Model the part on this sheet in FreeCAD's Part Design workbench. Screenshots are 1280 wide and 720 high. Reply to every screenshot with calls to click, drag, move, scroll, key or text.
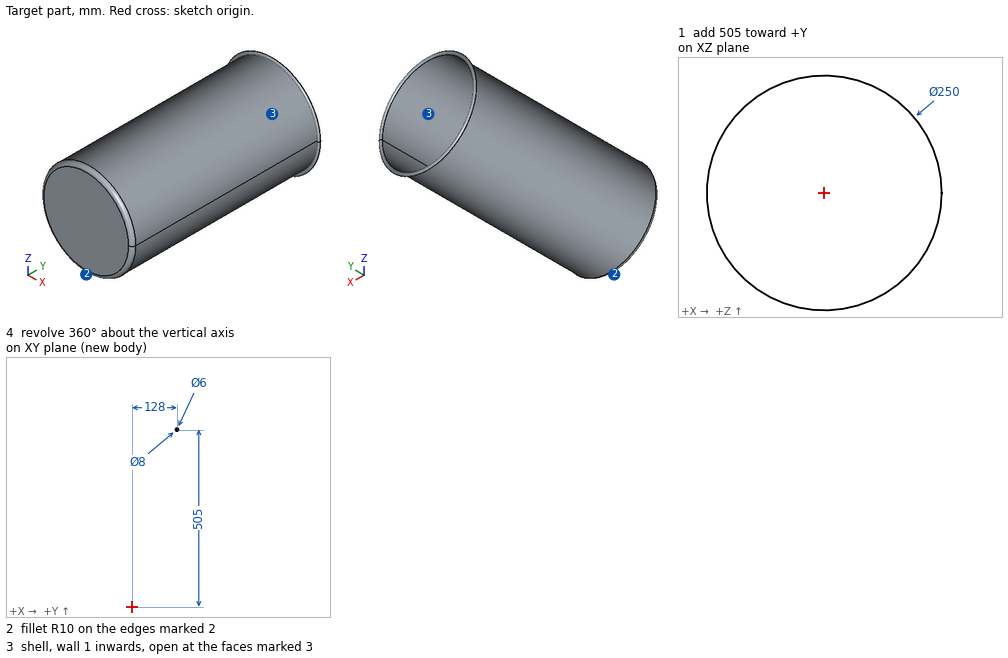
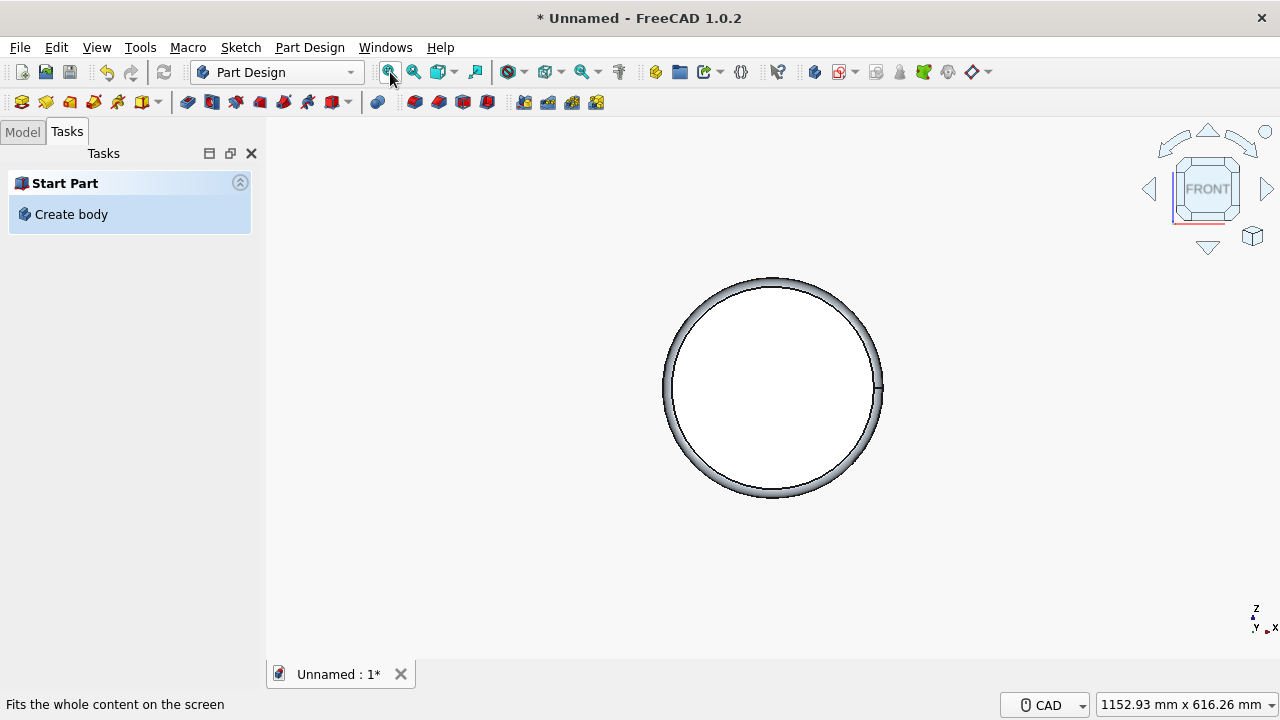
key(3)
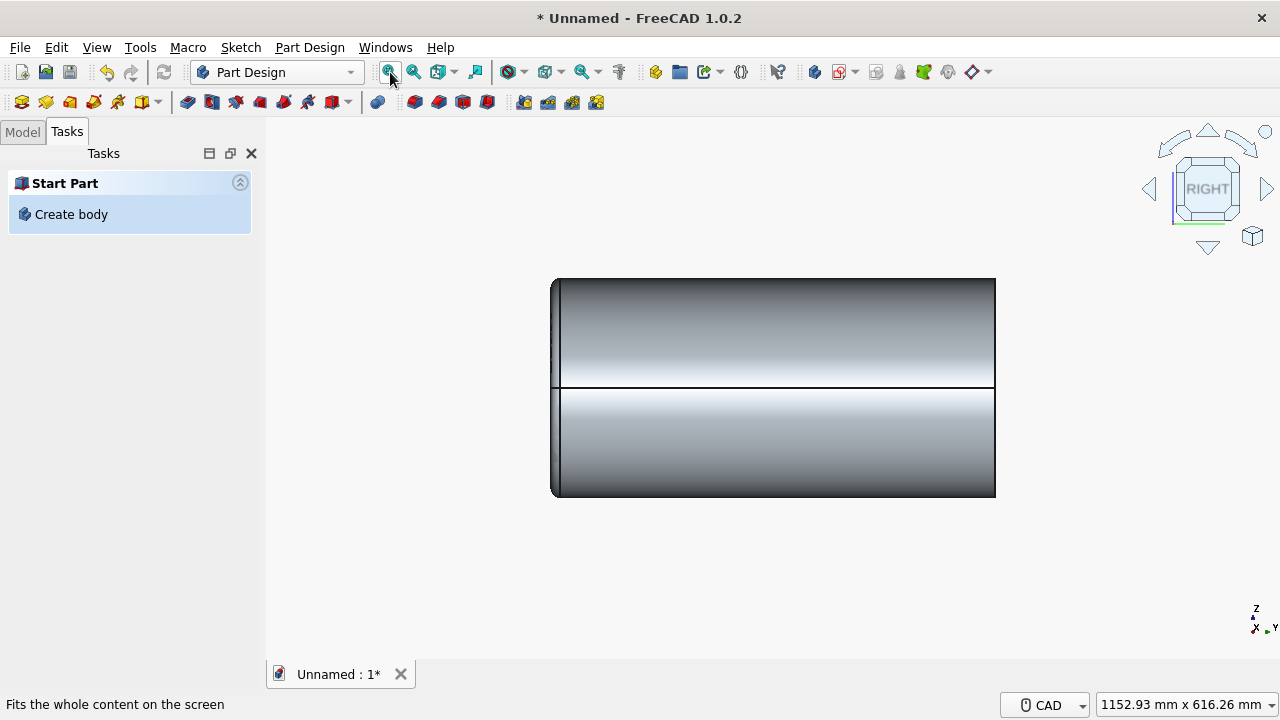
click(390, 72)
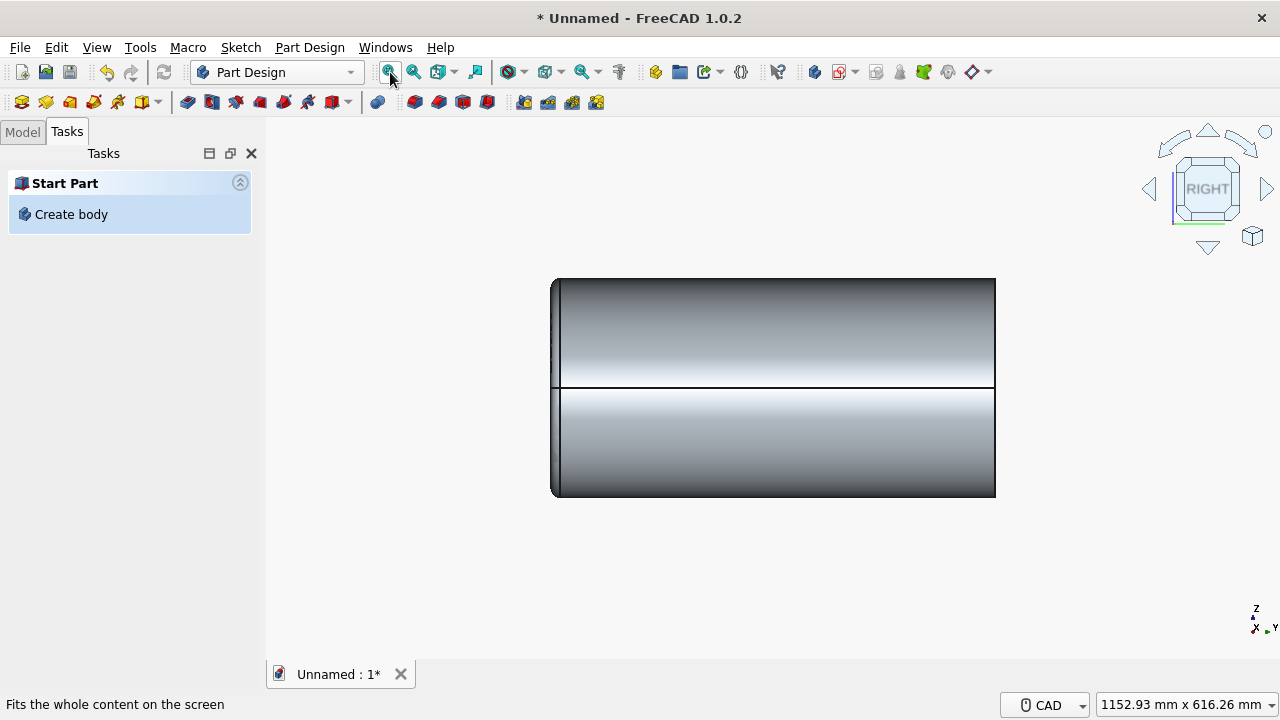
key(5)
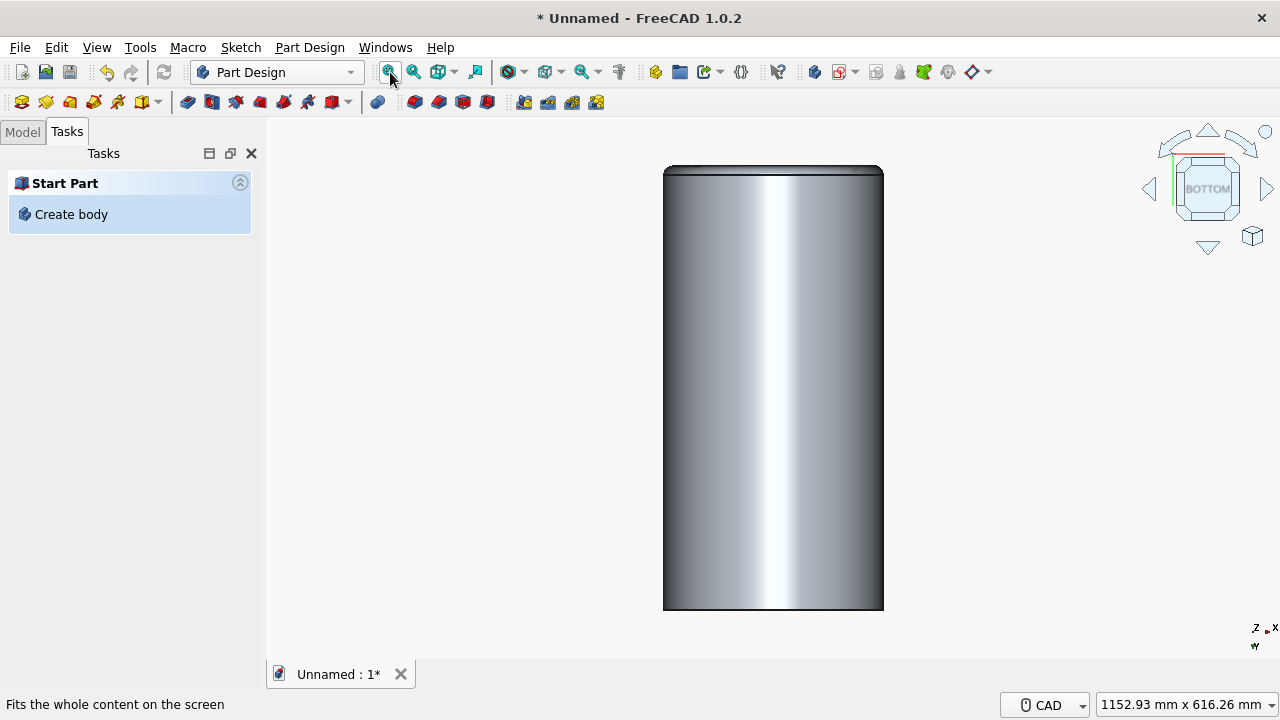
key(4)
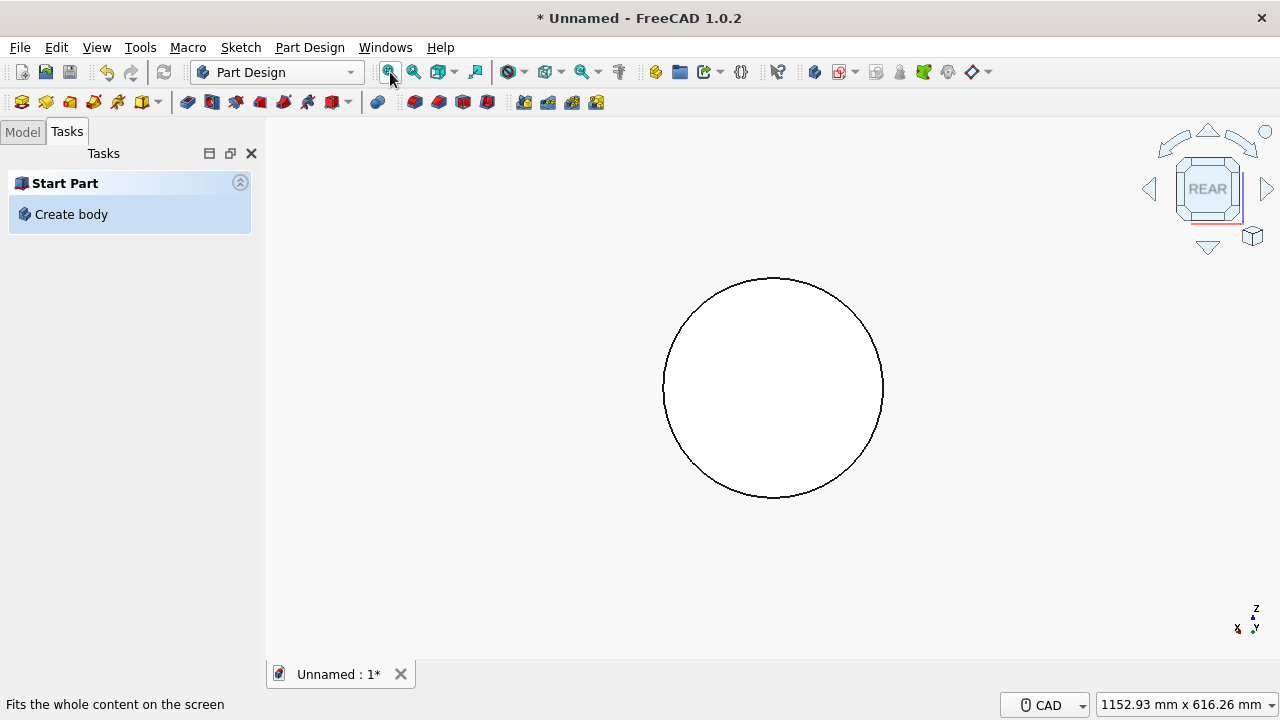
click(390, 72)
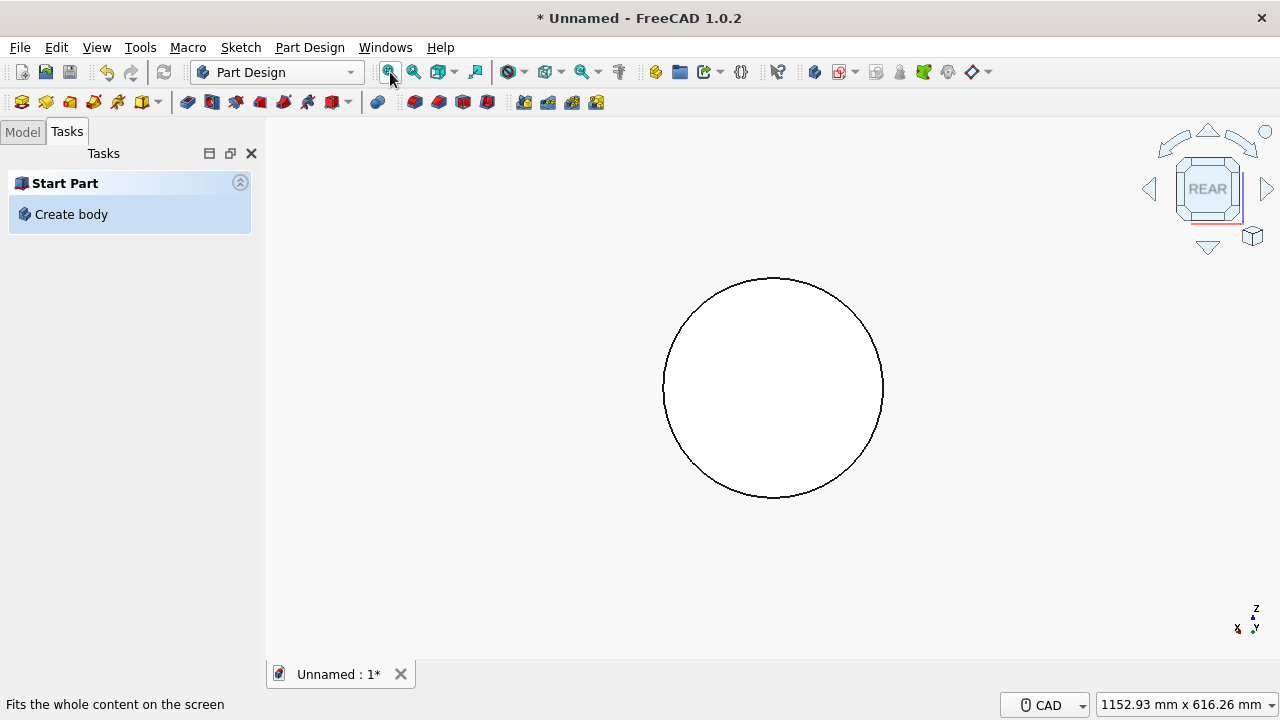
click(773, 387)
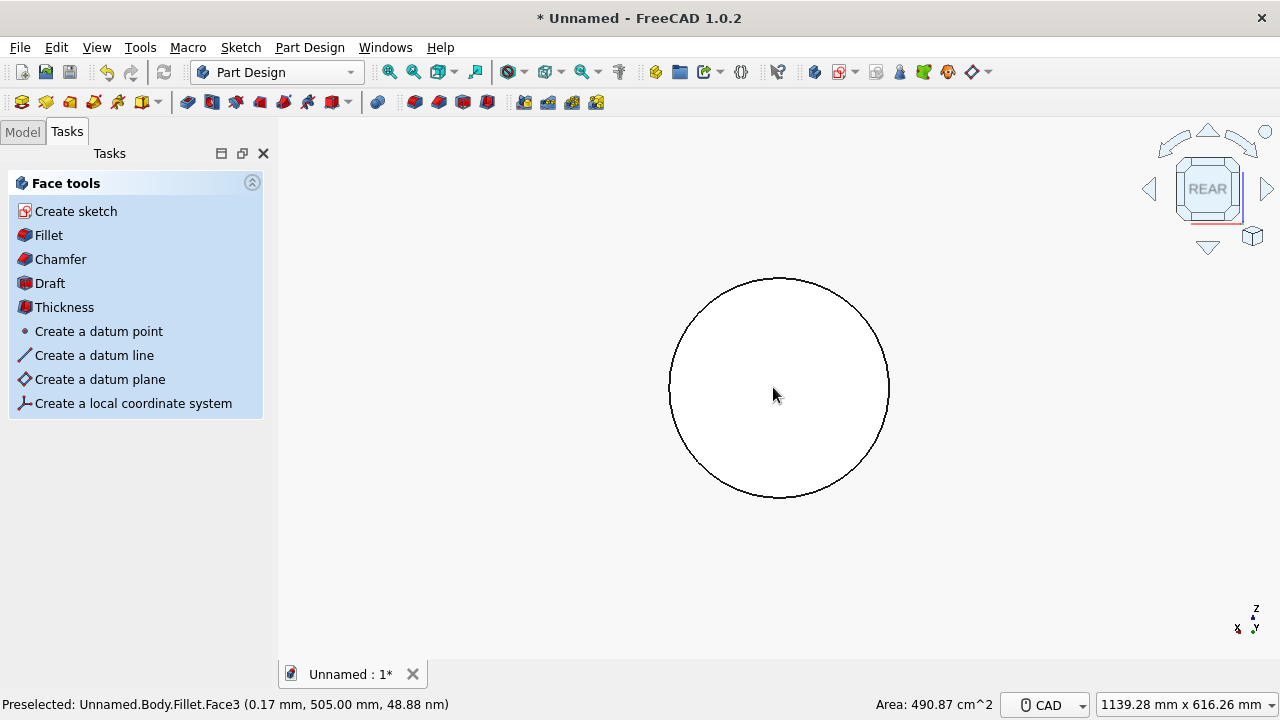
click(488, 102)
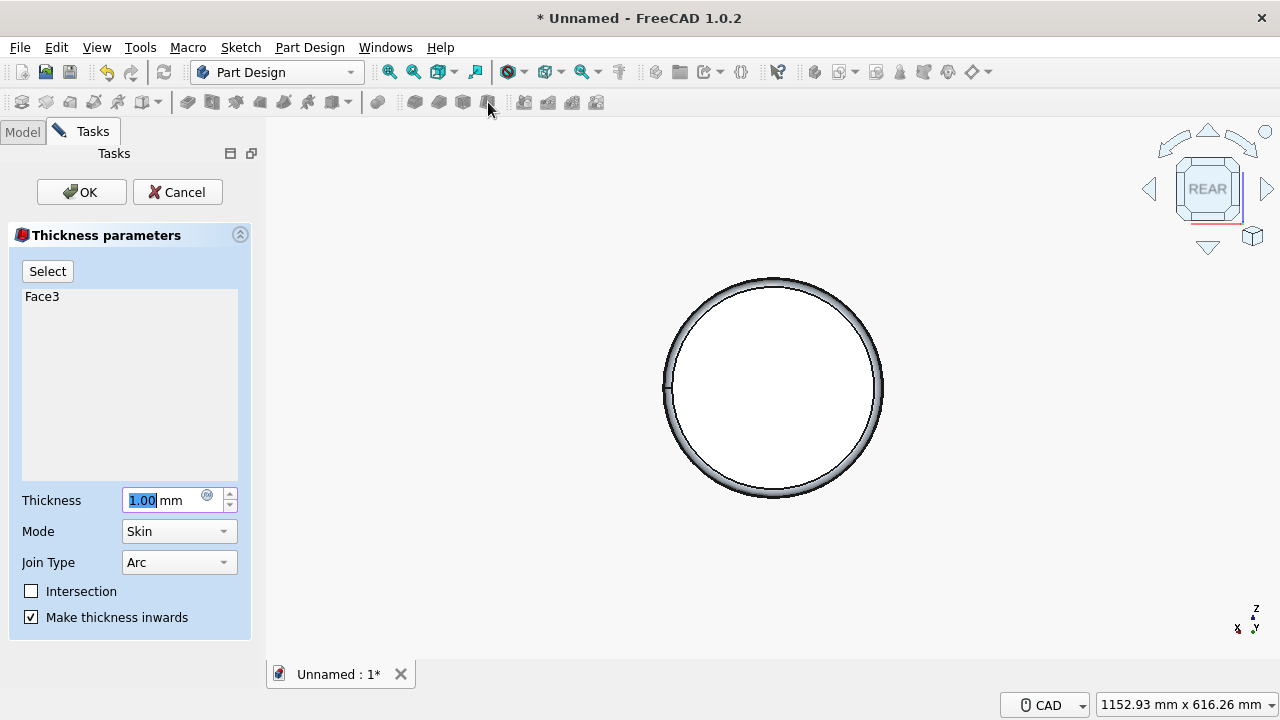
text(1)
key(Tab)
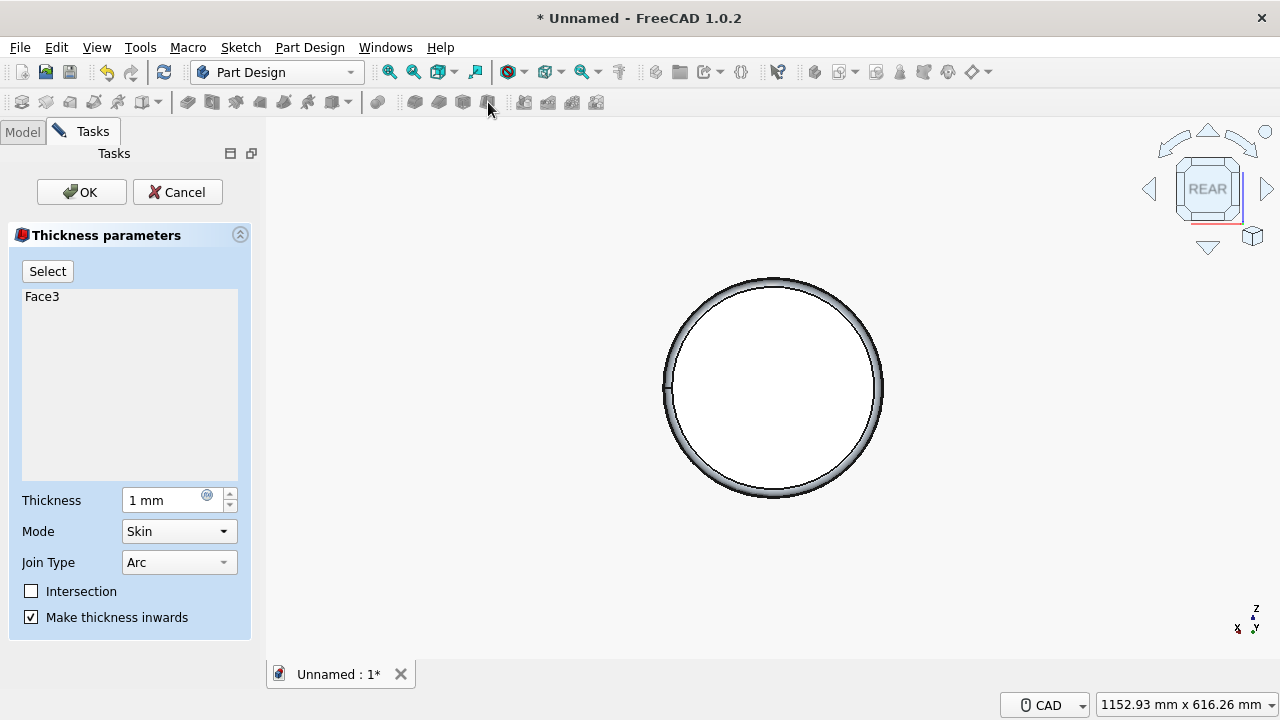
click(180, 562)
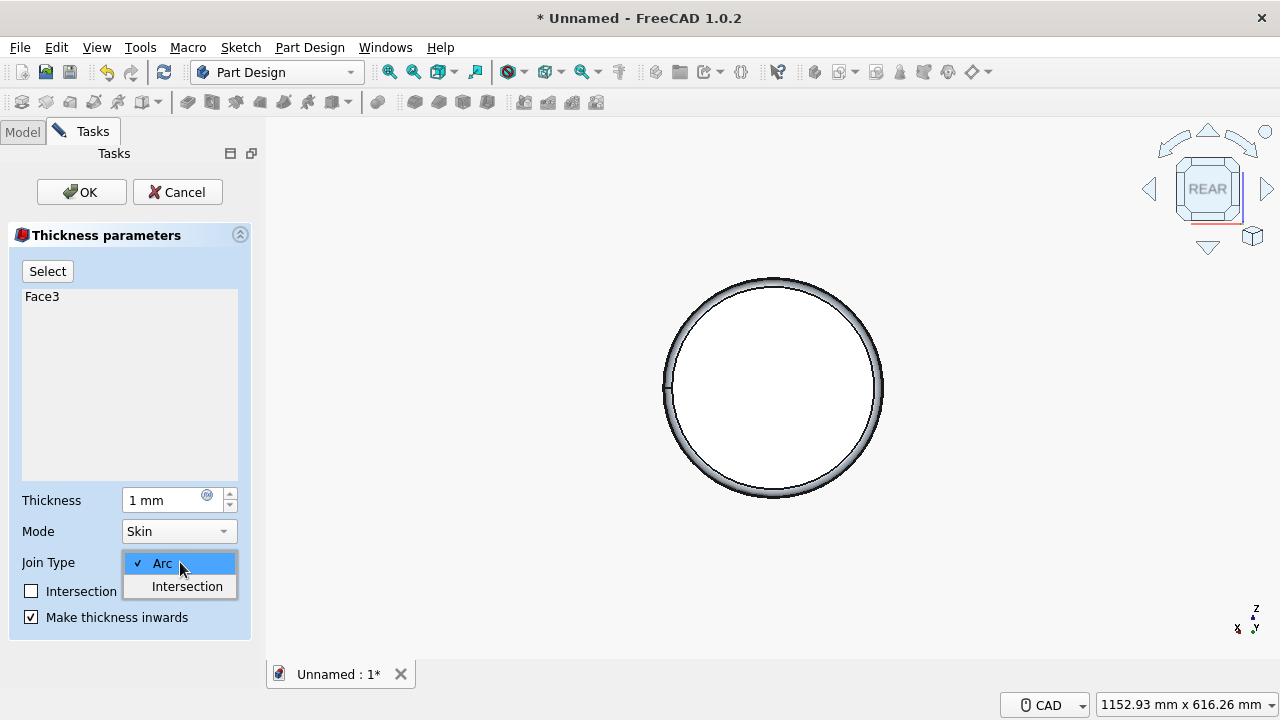
click(179, 586)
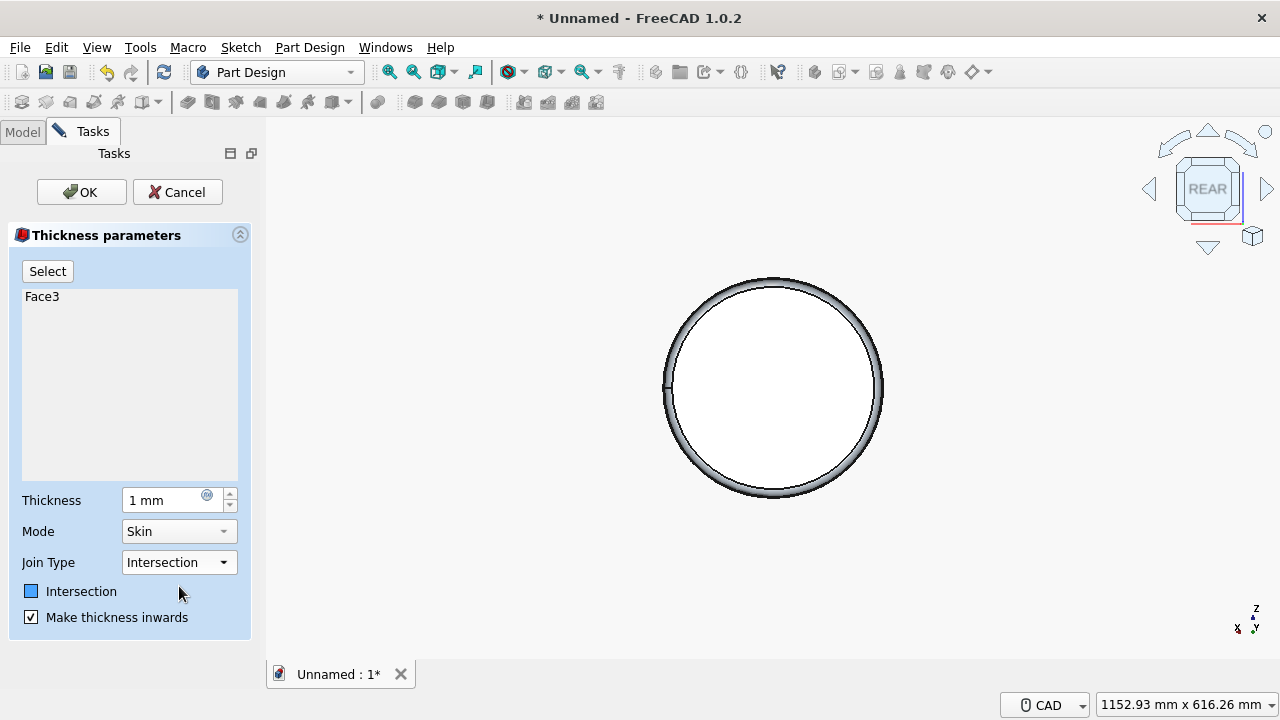
click(82, 192)